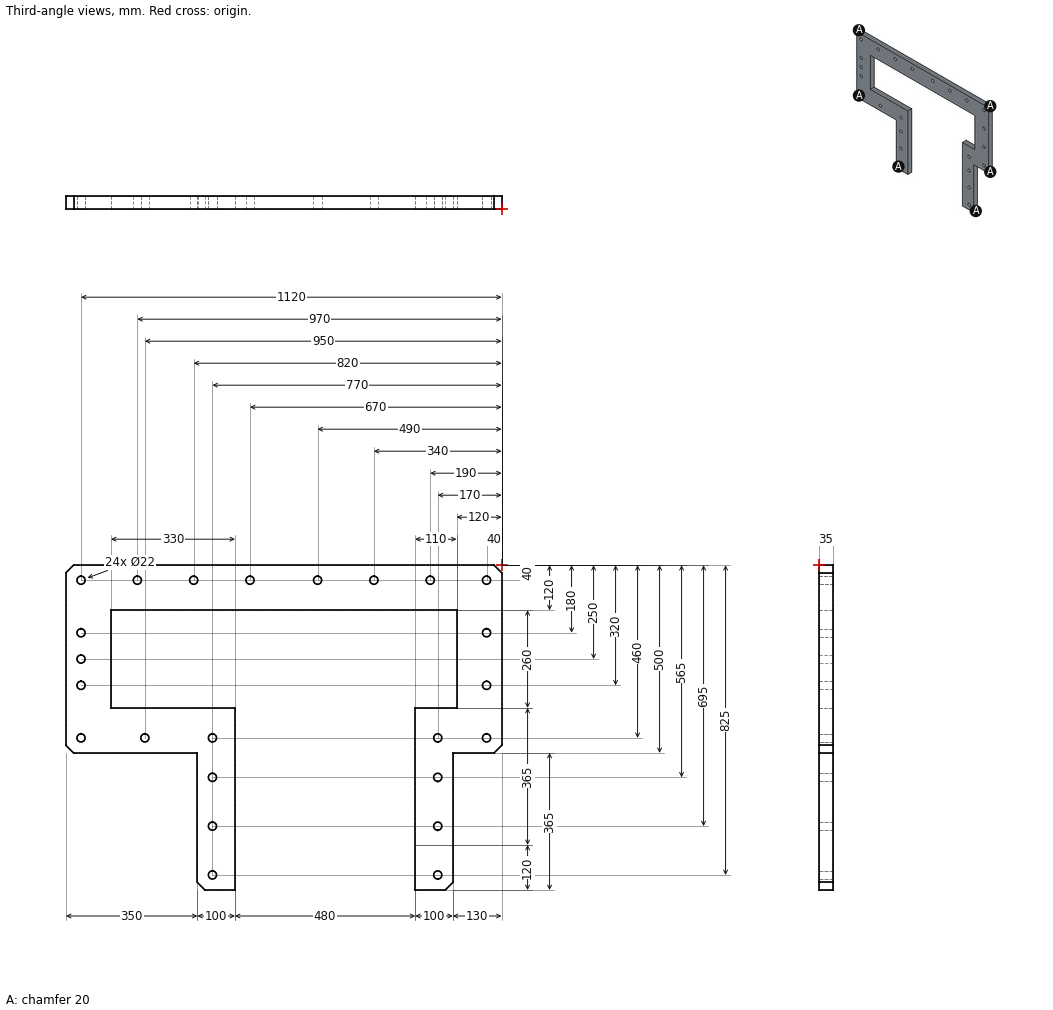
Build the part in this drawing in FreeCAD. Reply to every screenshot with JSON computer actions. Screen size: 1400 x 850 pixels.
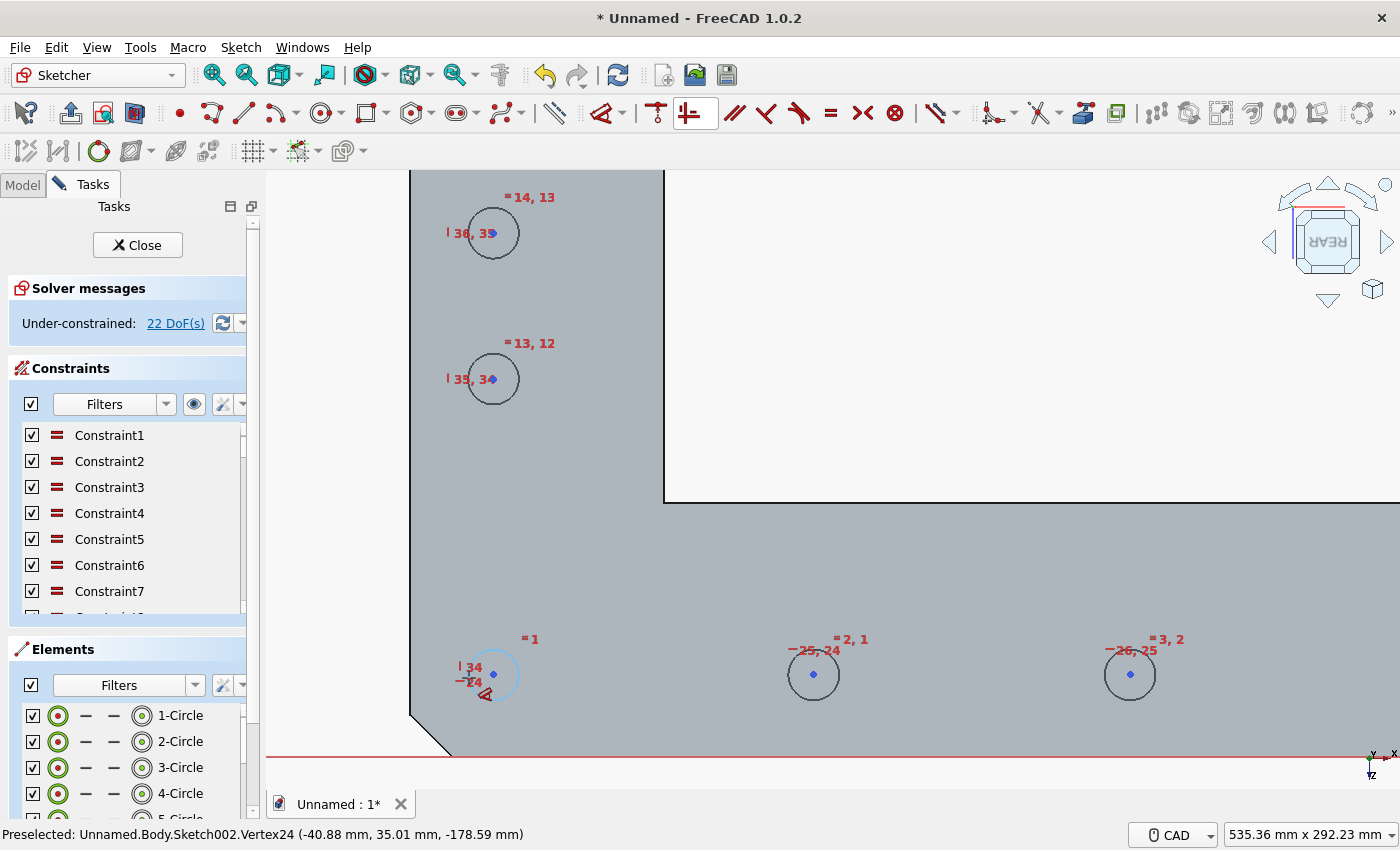
{"action": "left_click", "coordinate": [468, 674]}
{"action": "left_click", "coordinate": [436, 673]}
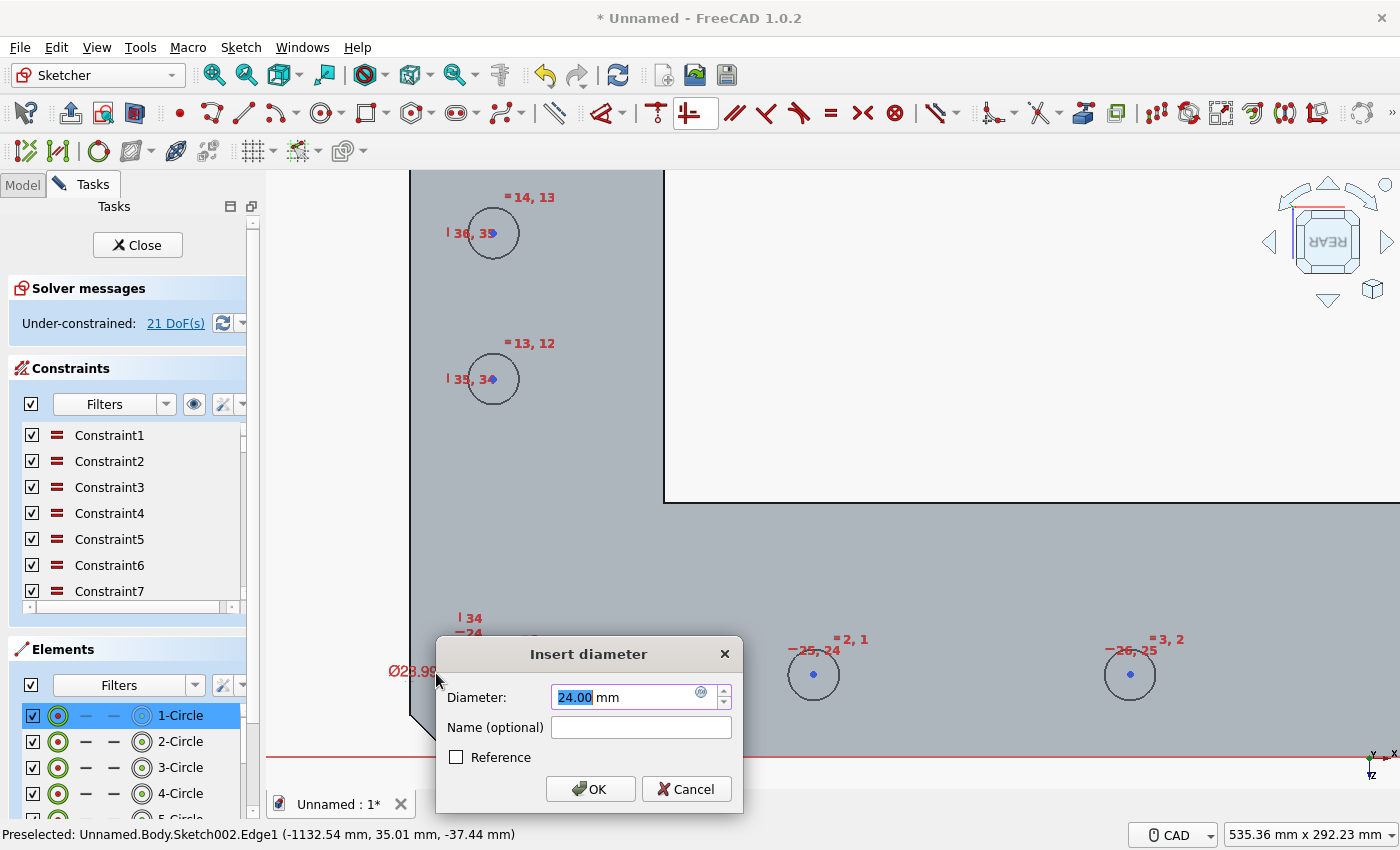
{"action": "type", "text": "22"}
{"action": "key", "text": "Return"}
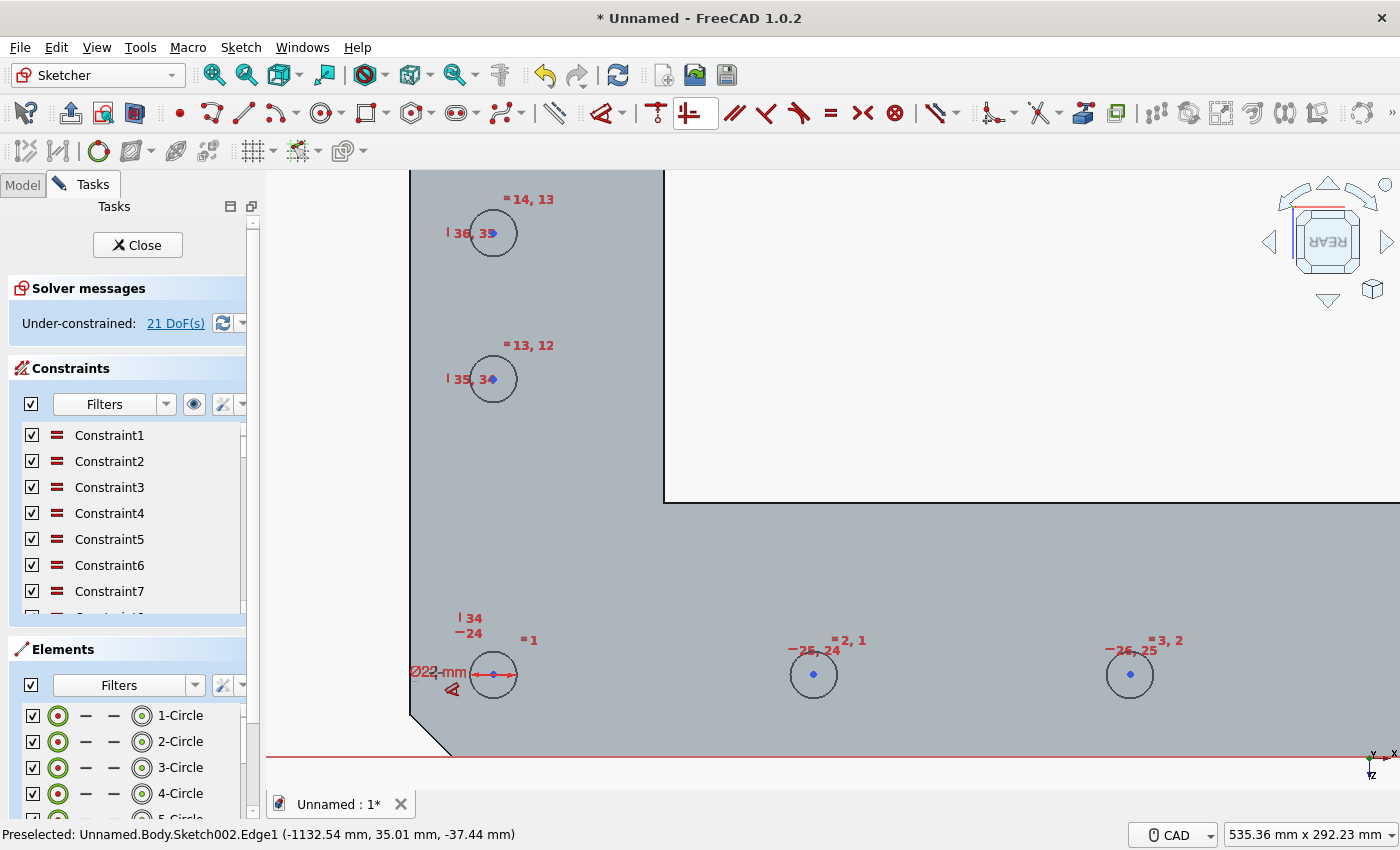
{"action": "left_click", "coordinate": [493, 675]}
{"action": "left_click", "coordinate": [459, 716]}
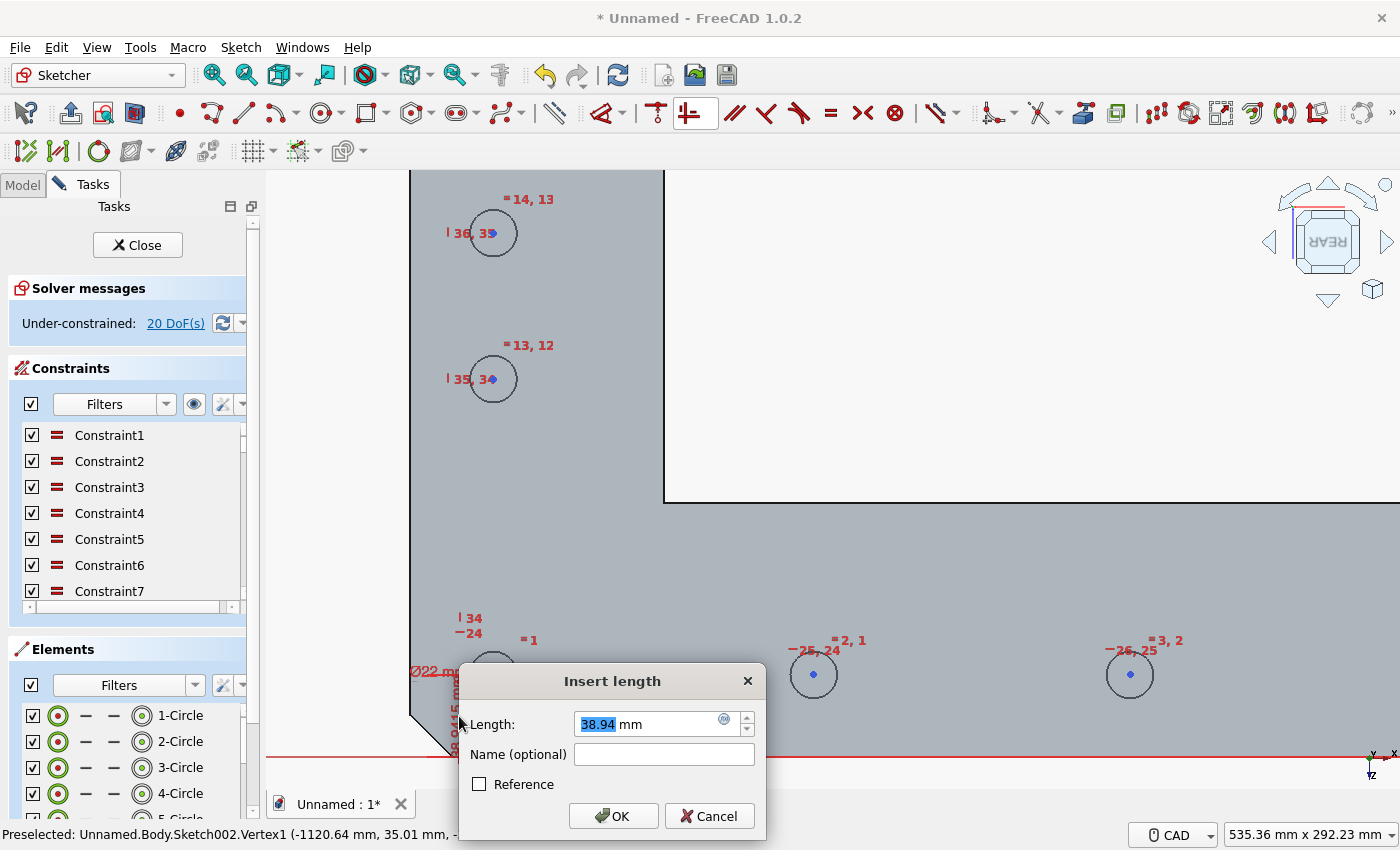
{"action": "type", "text": "40"}
{"action": "key", "text": "Return"}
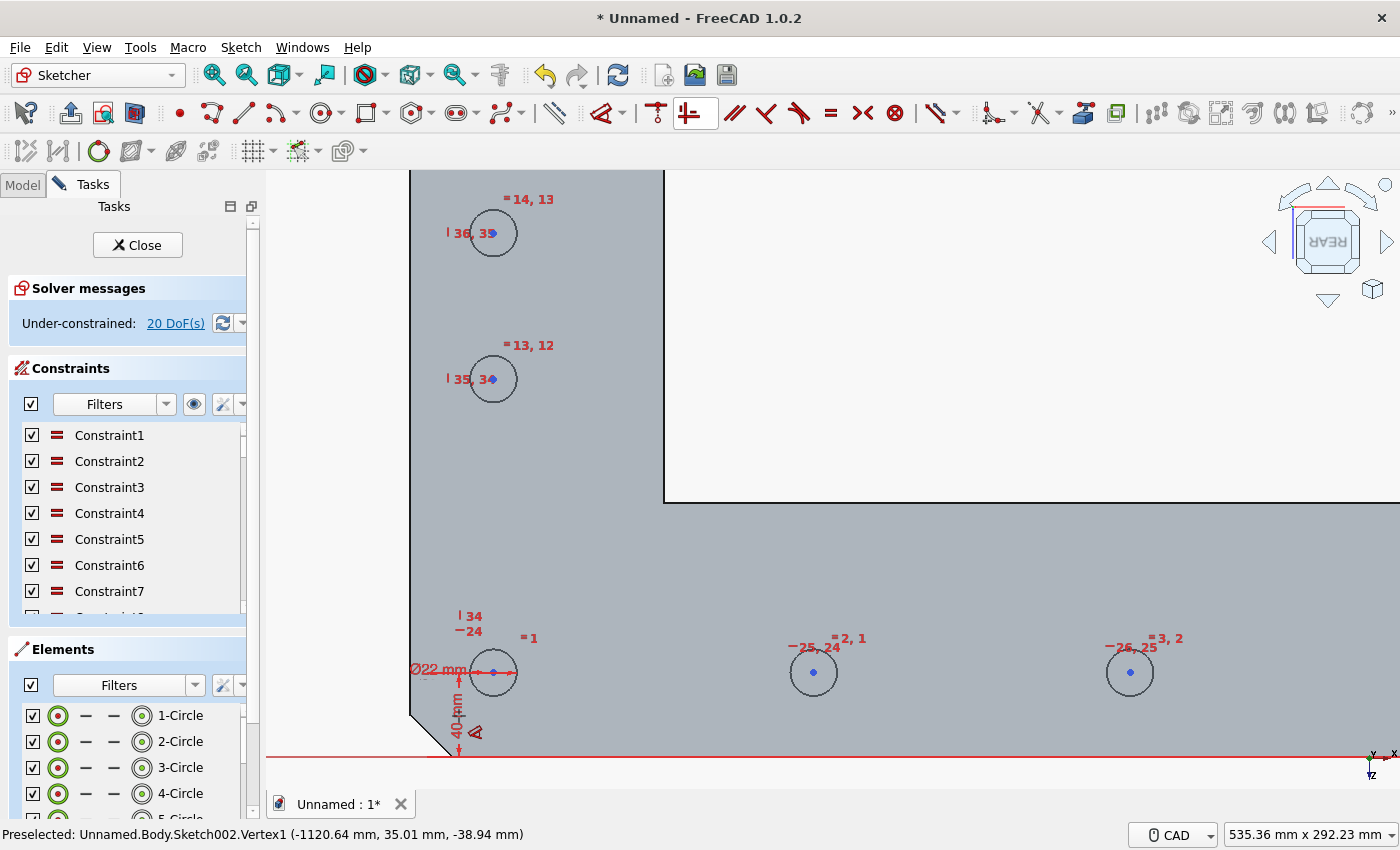
{"action": "scroll", "coordinate": [468, 678], "scroll_direction": "down", "scroll_amount": 7}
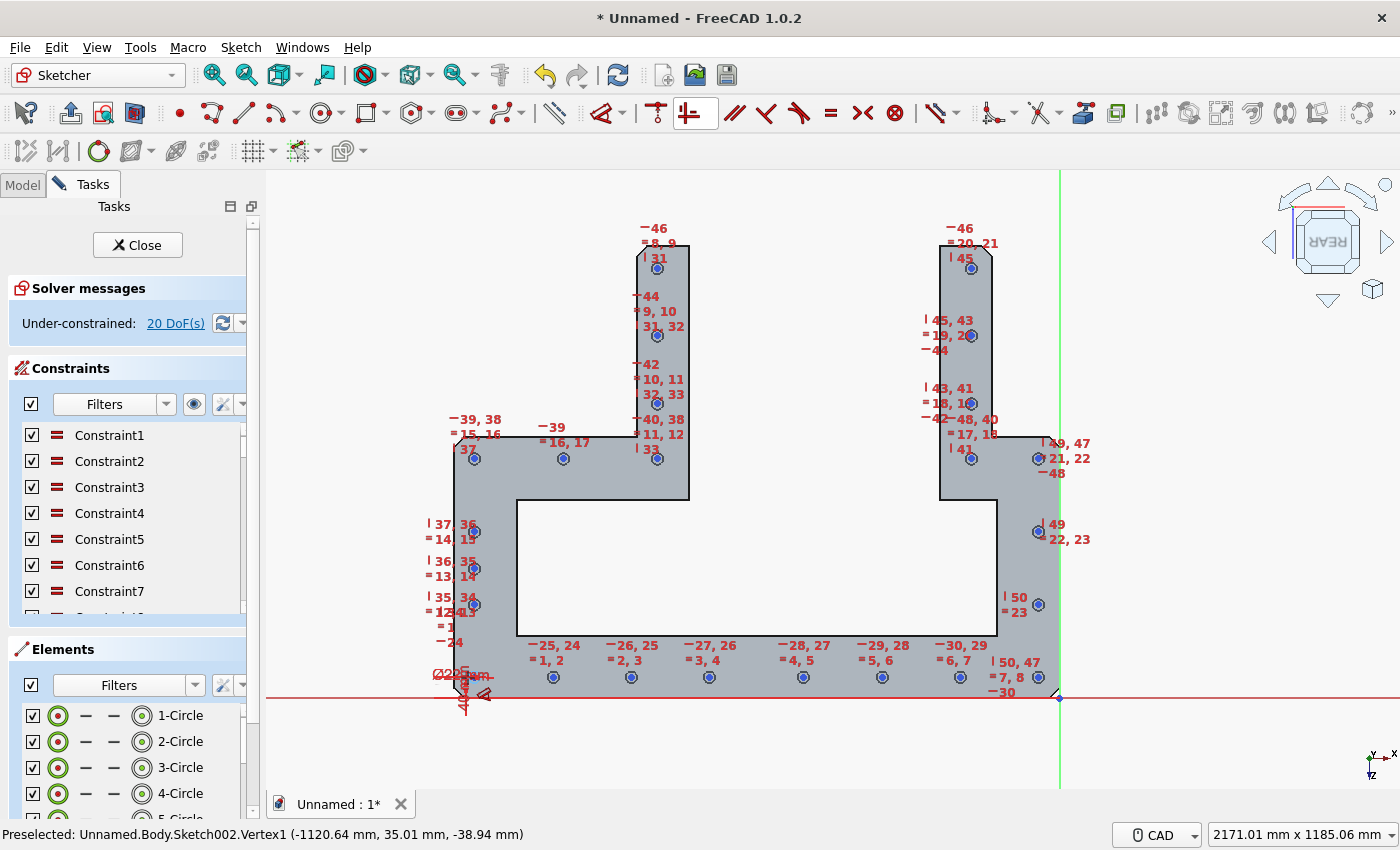
{"action": "scroll", "coordinate": [1038, 677], "scroll_direction": "up", "scroll_amount": 4}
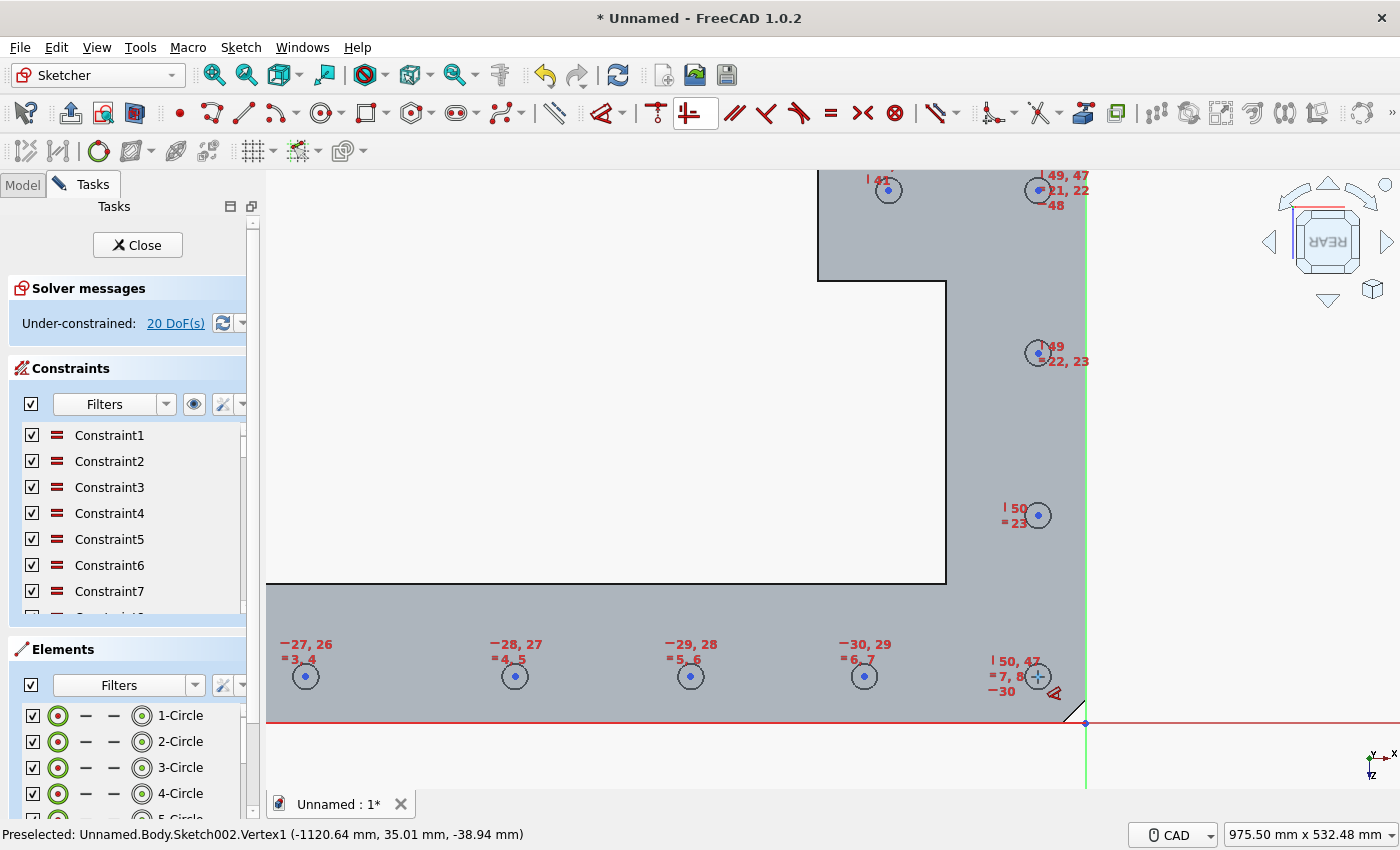
{"action": "left_click", "coordinate": [1038, 677]}
{"action": "left_click", "coordinate": [1062, 757]}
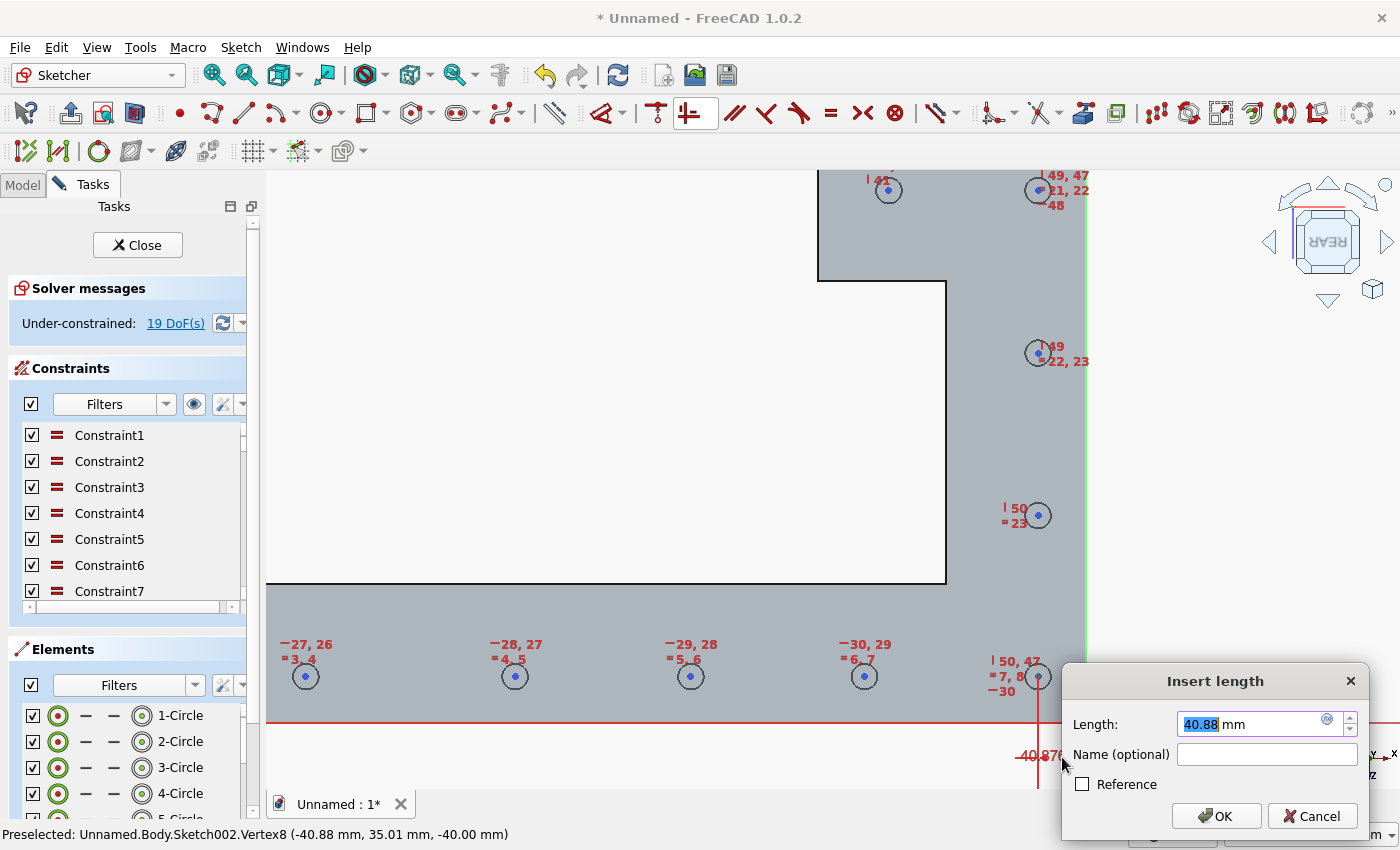
{"action": "type", "text": "40"}
{"action": "key", "text": "Return"}